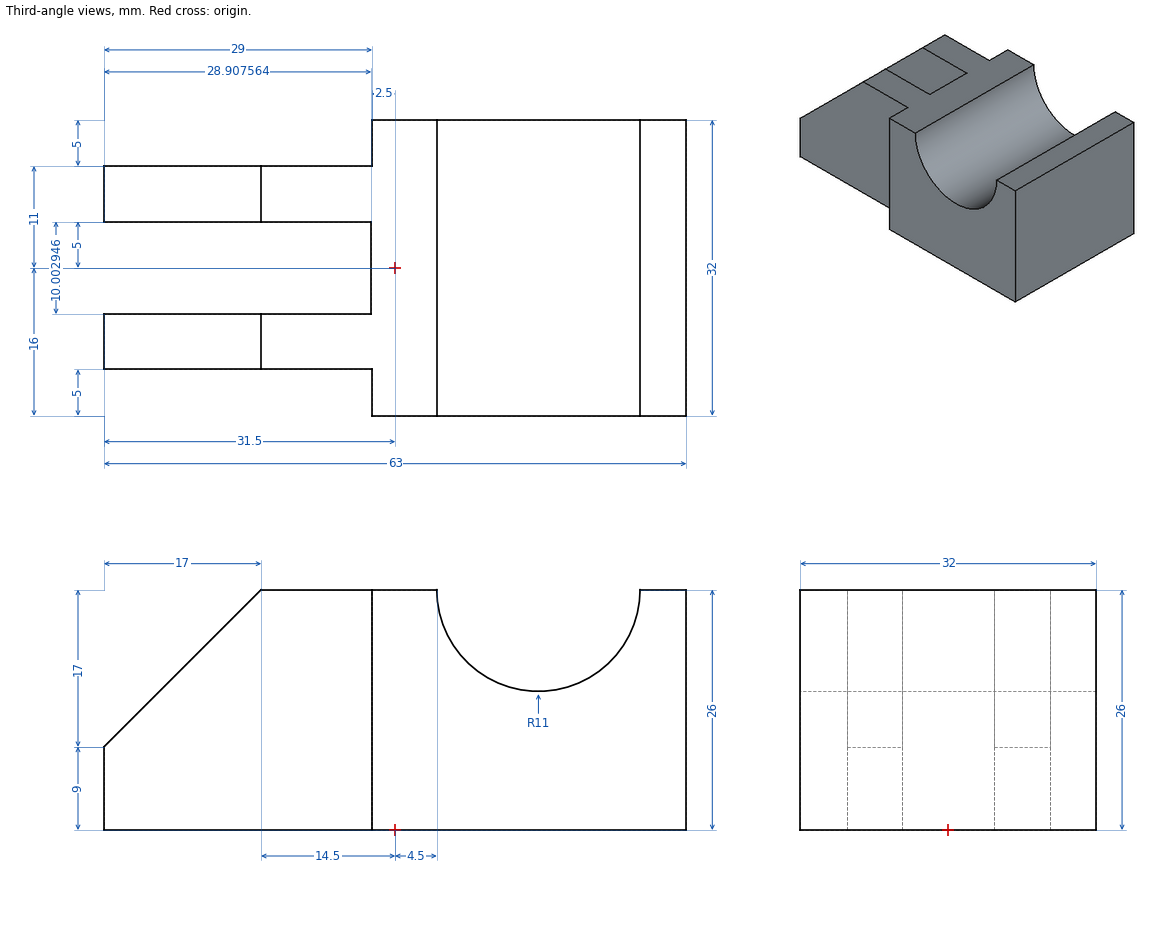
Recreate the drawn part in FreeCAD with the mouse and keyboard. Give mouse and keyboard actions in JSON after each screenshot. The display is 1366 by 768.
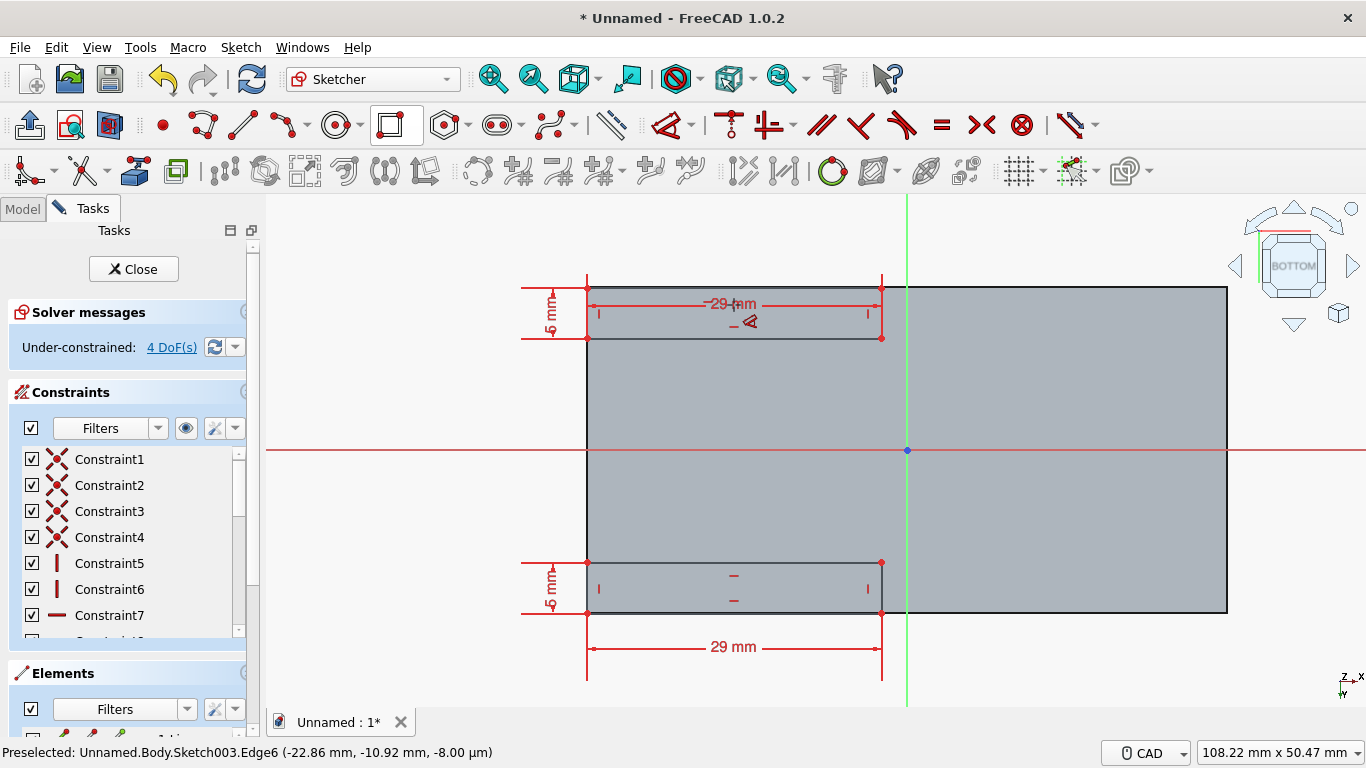
{"action": "left_click", "coordinate": [587, 563]}
{"action": "left_click", "coordinate": [553, 507]}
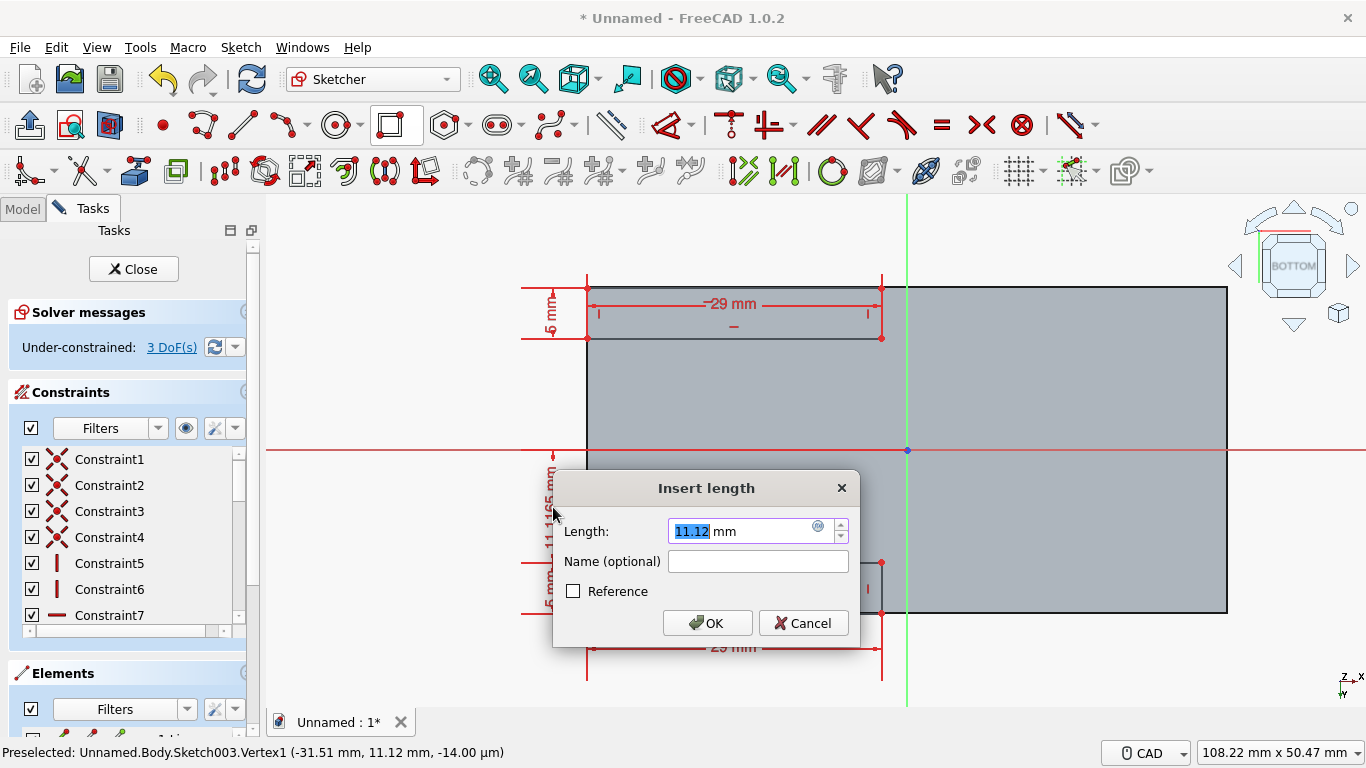
{"action": "type", "text": "11"}
{"action": "key", "text": "Return"}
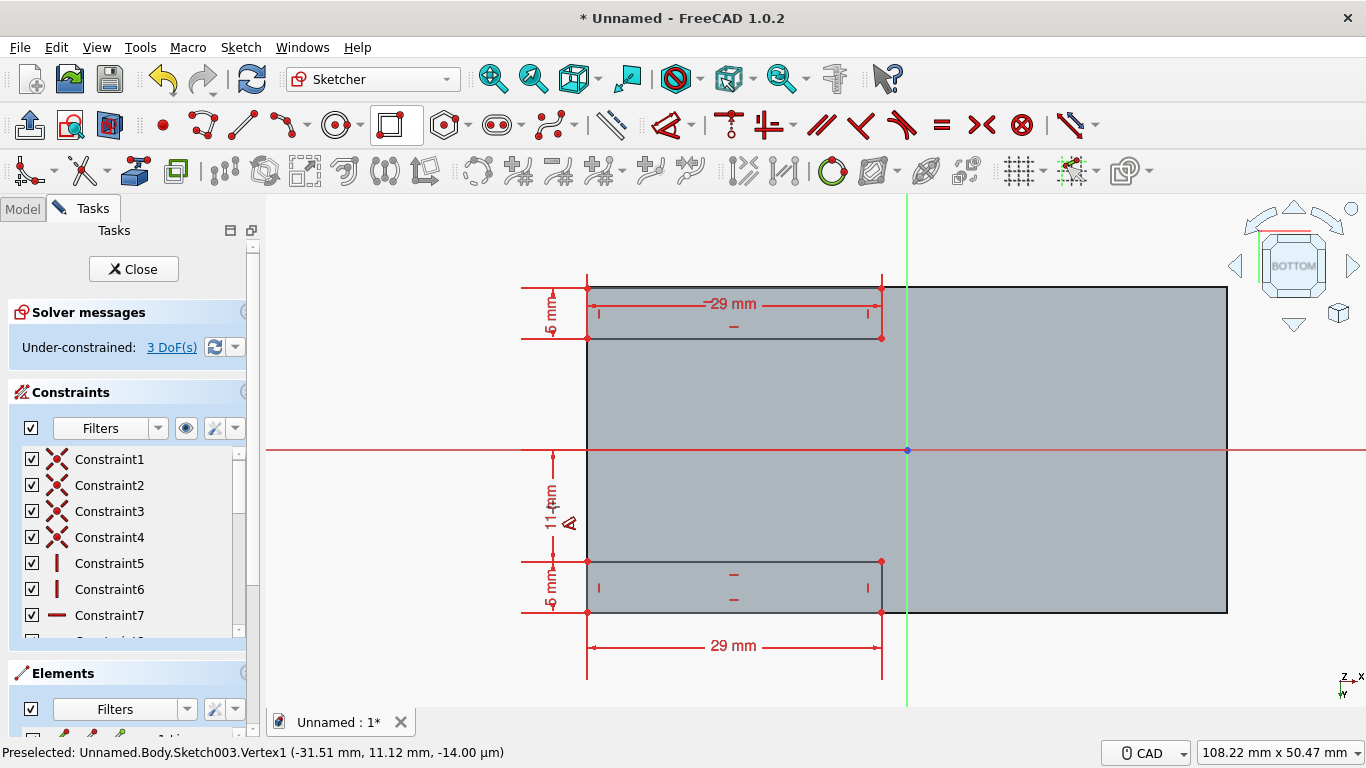
{"action": "left_click", "coordinate": [587, 288]}
{"action": "left_click", "coordinate": [553, 369]}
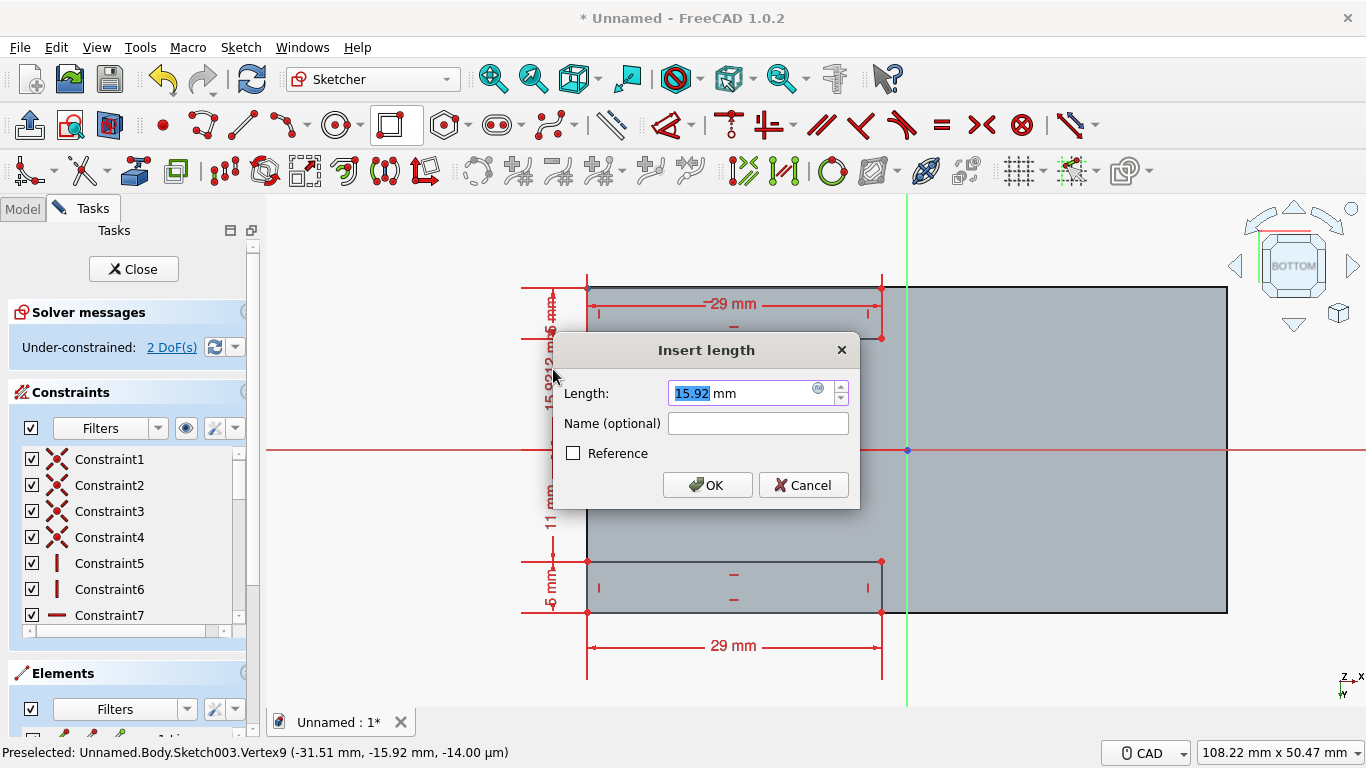
{"action": "type", "text": "16"}
{"action": "key", "text": "Return"}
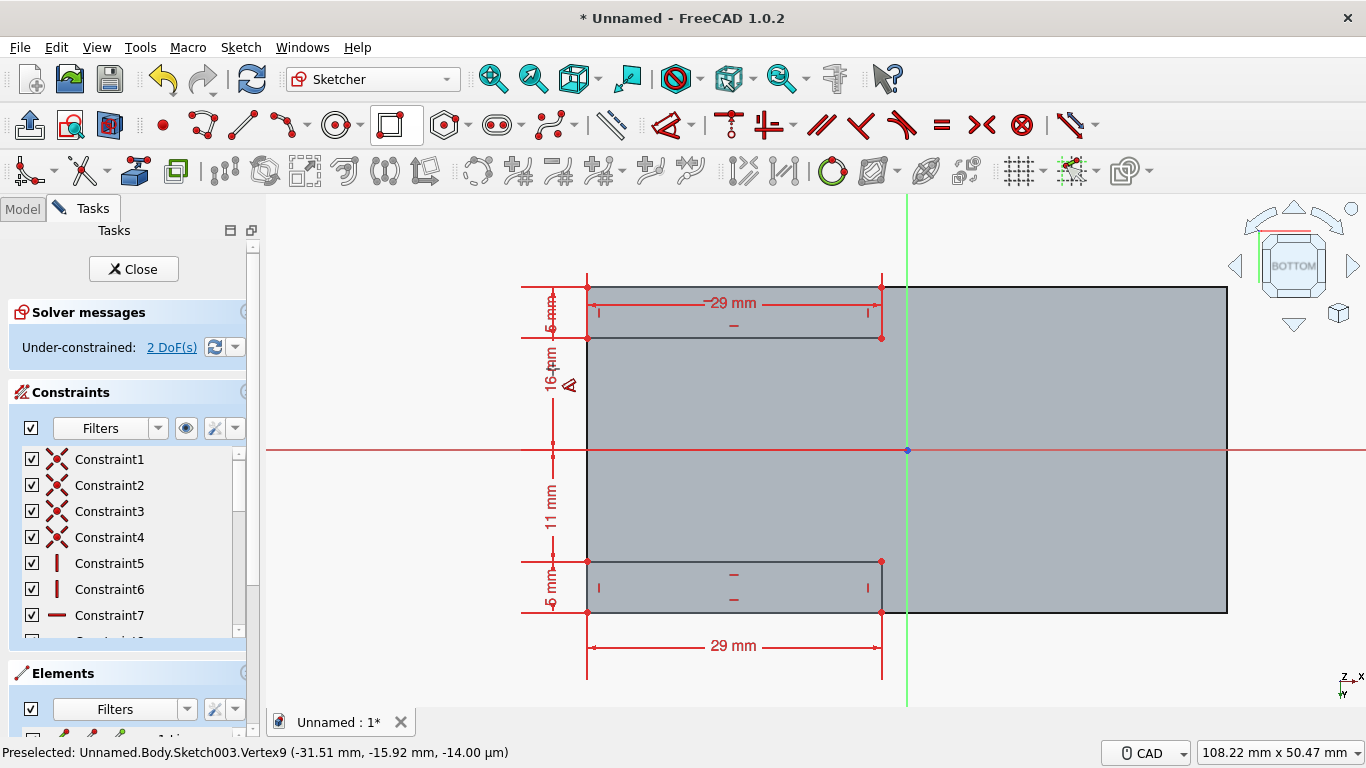
{"action": "scroll", "coordinate": [882, 613], "scroll_direction": "up", "scroll_amount": 3}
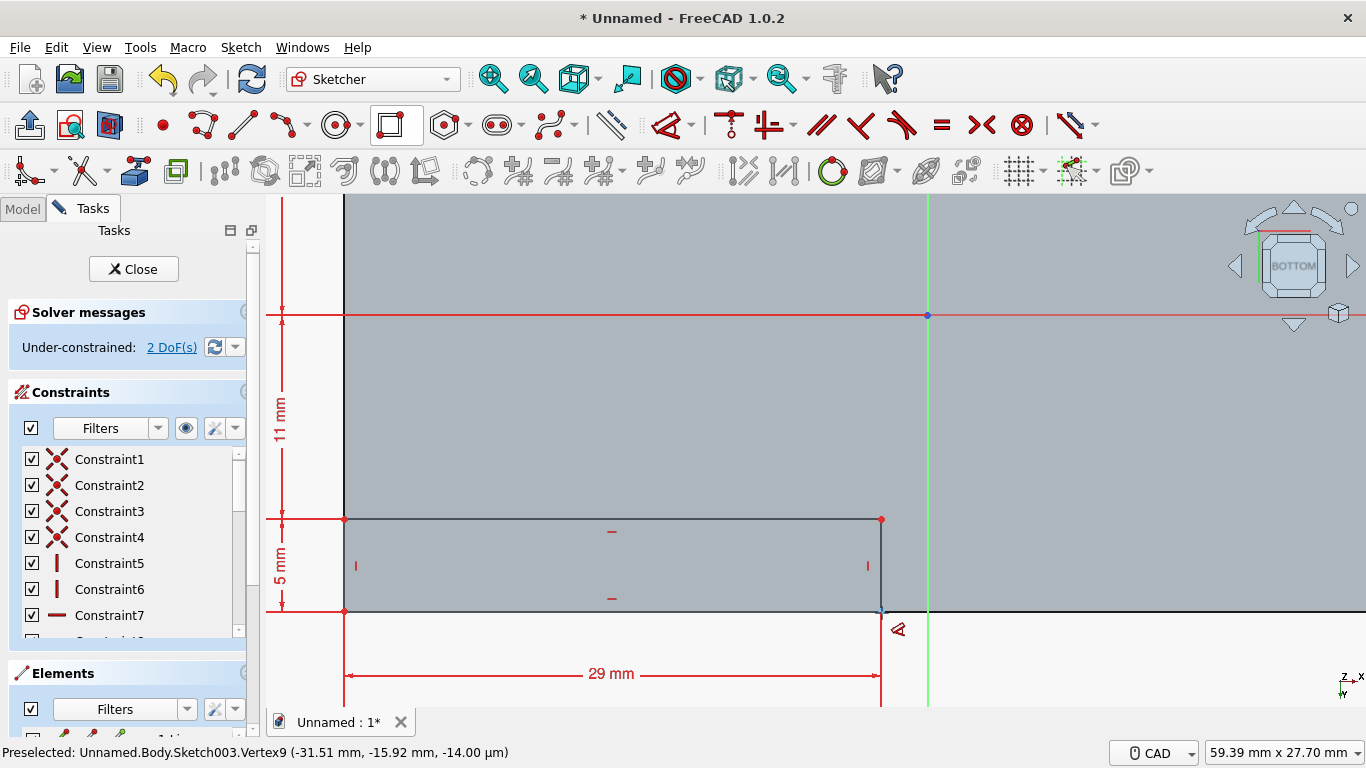
{"action": "left_click", "coordinate": [881, 612]}
{"action": "left_click", "coordinate": [904, 646]}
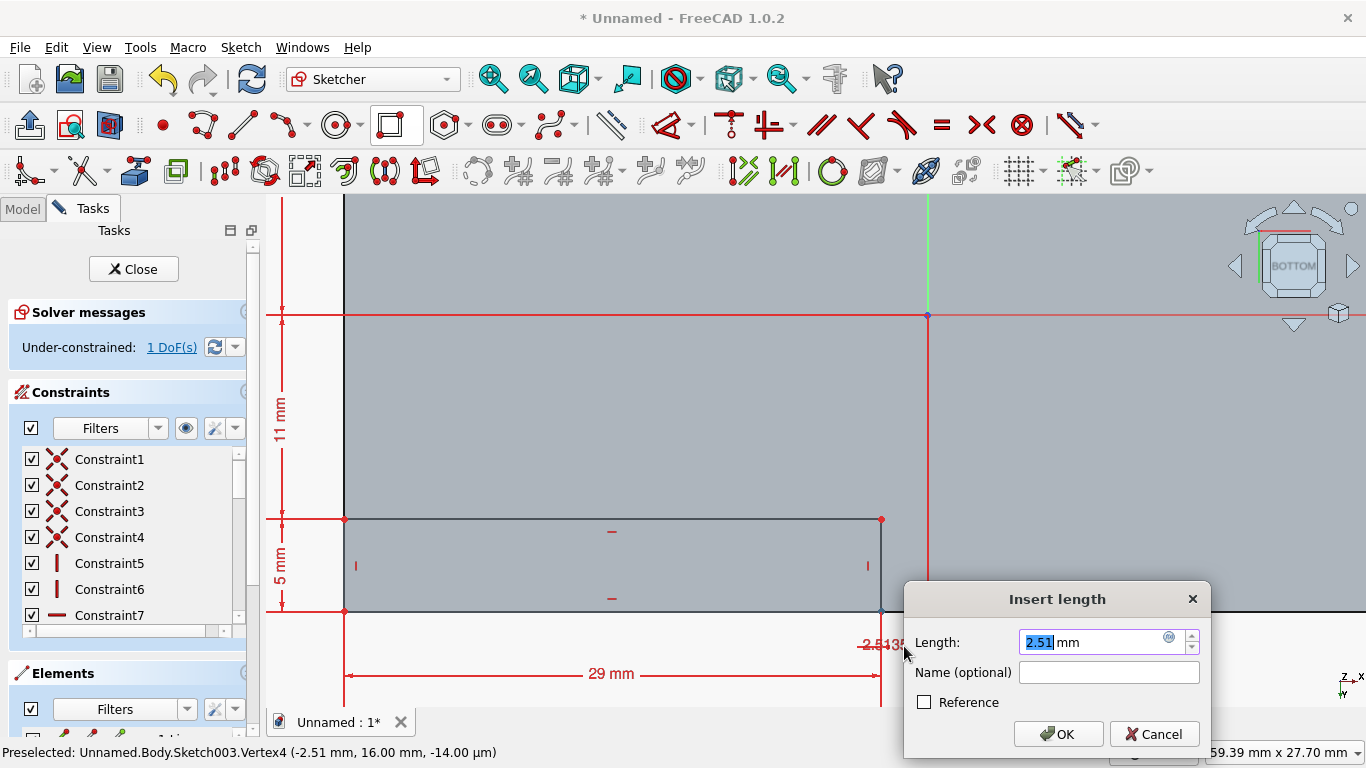
{"action": "type", "text": "2.5"}
{"action": "key", "text": "Return"}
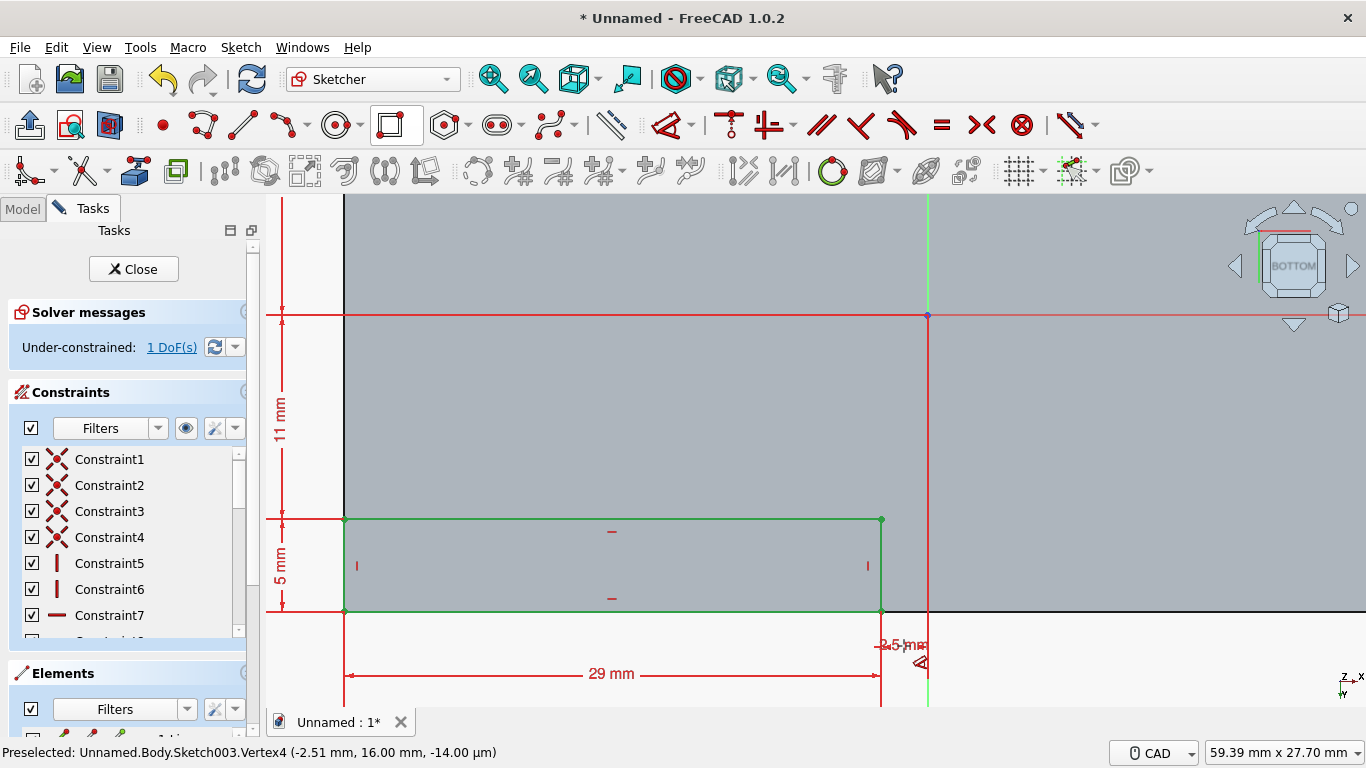
{"action": "scroll", "coordinate": [883, 615], "scroll_direction": "down", "scroll_amount": 3}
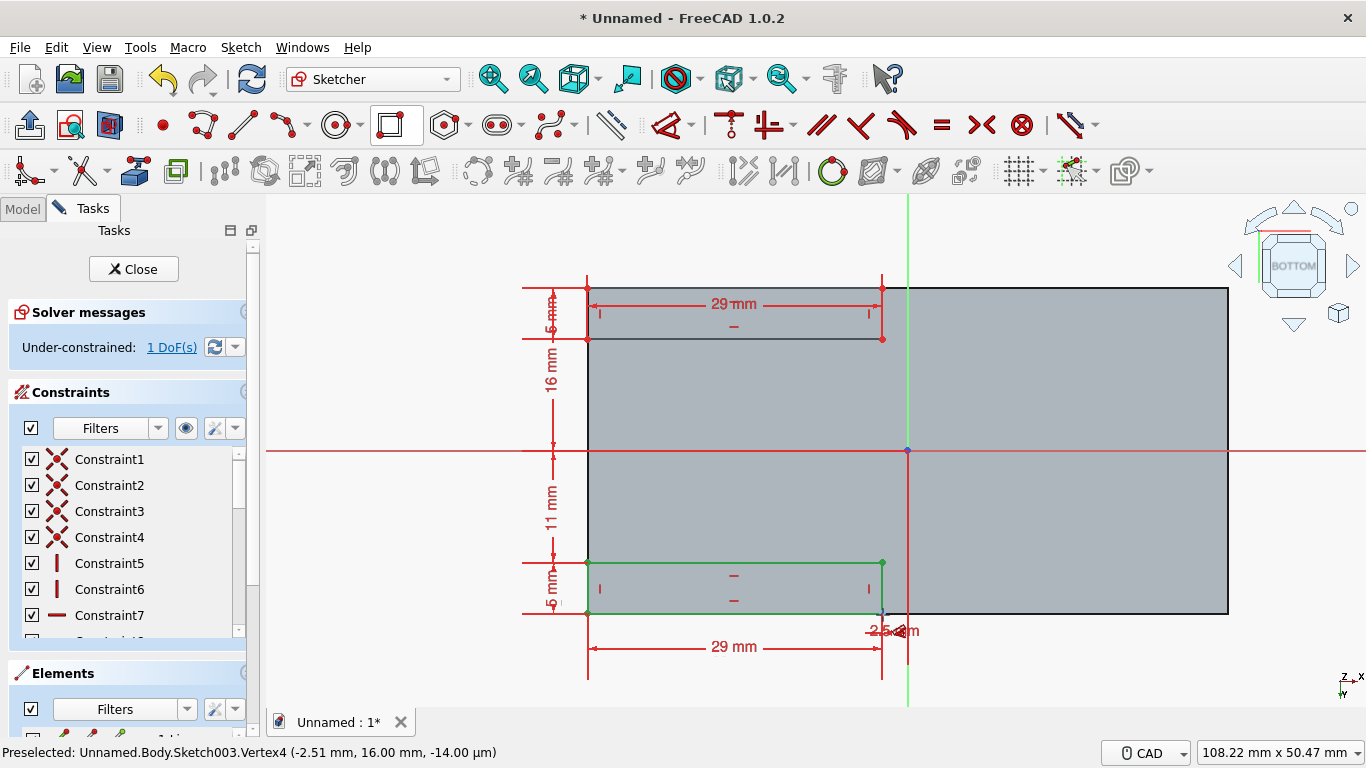
{"action": "scroll", "coordinate": [882, 339], "scroll_direction": "up", "scroll_amount": 3}